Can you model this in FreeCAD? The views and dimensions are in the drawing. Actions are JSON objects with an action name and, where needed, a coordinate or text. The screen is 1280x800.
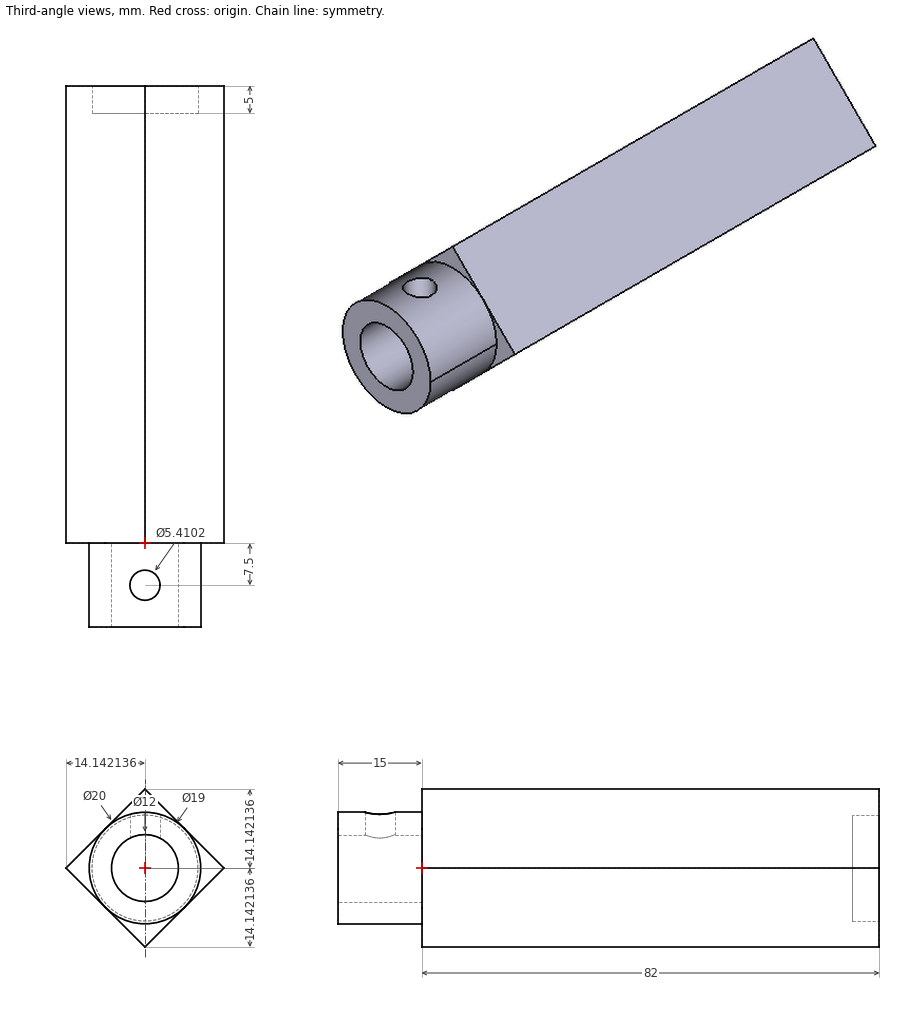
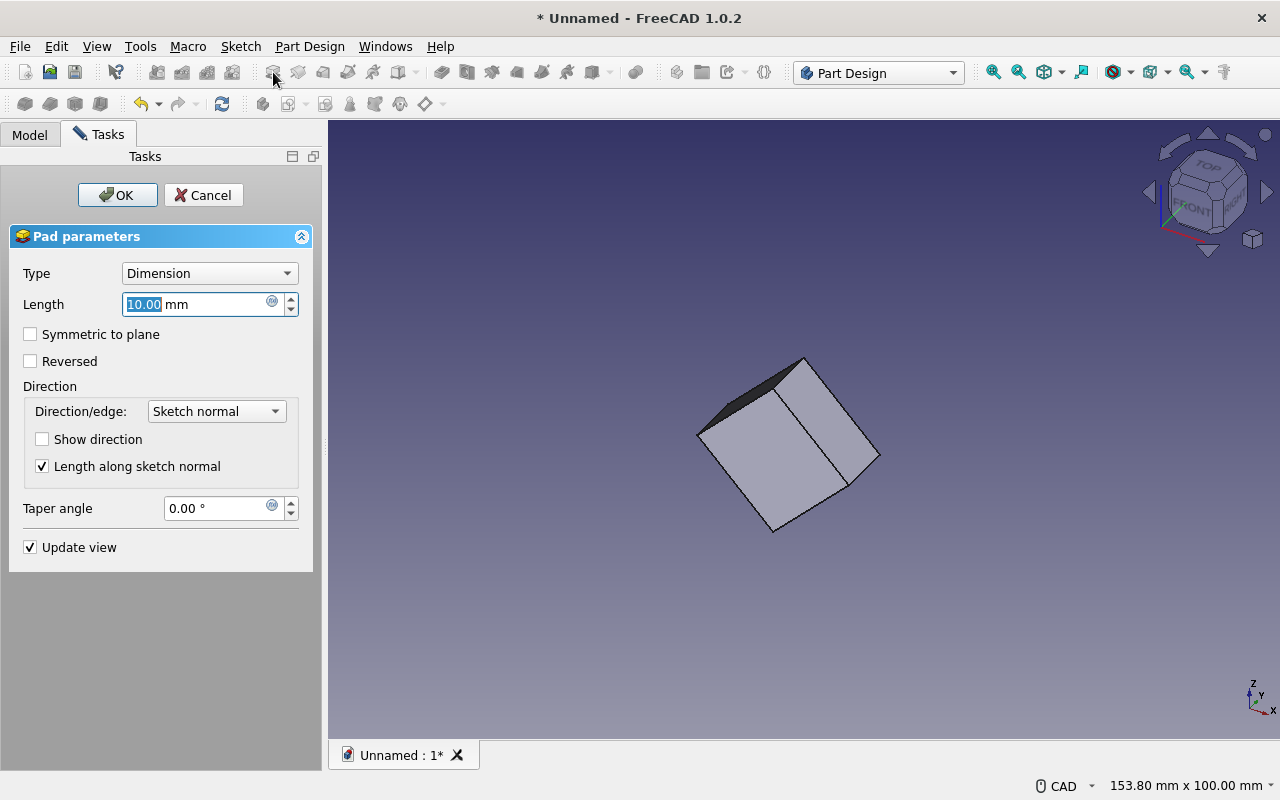
{"action": "type", "text": "82"}
{"action": "key", "text": "Tab"}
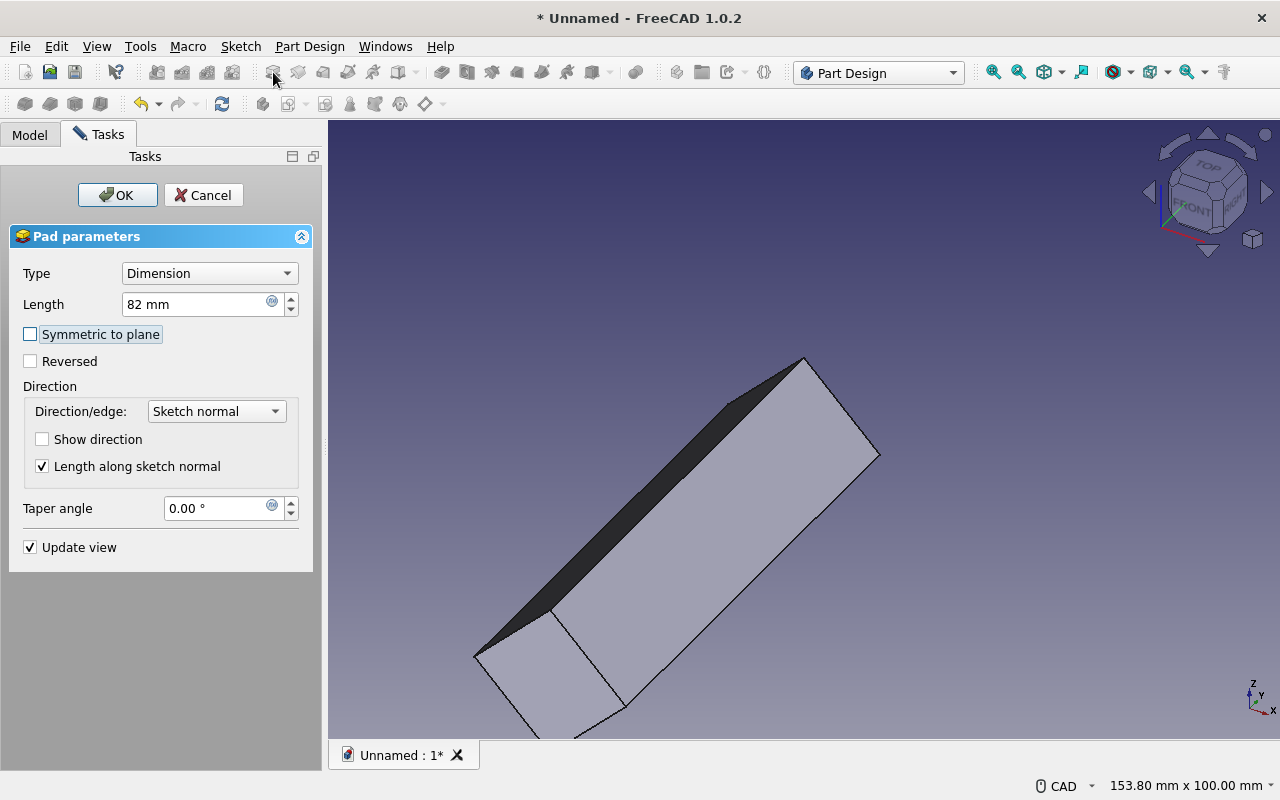
{"action": "left_click", "coordinate": [31, 361]}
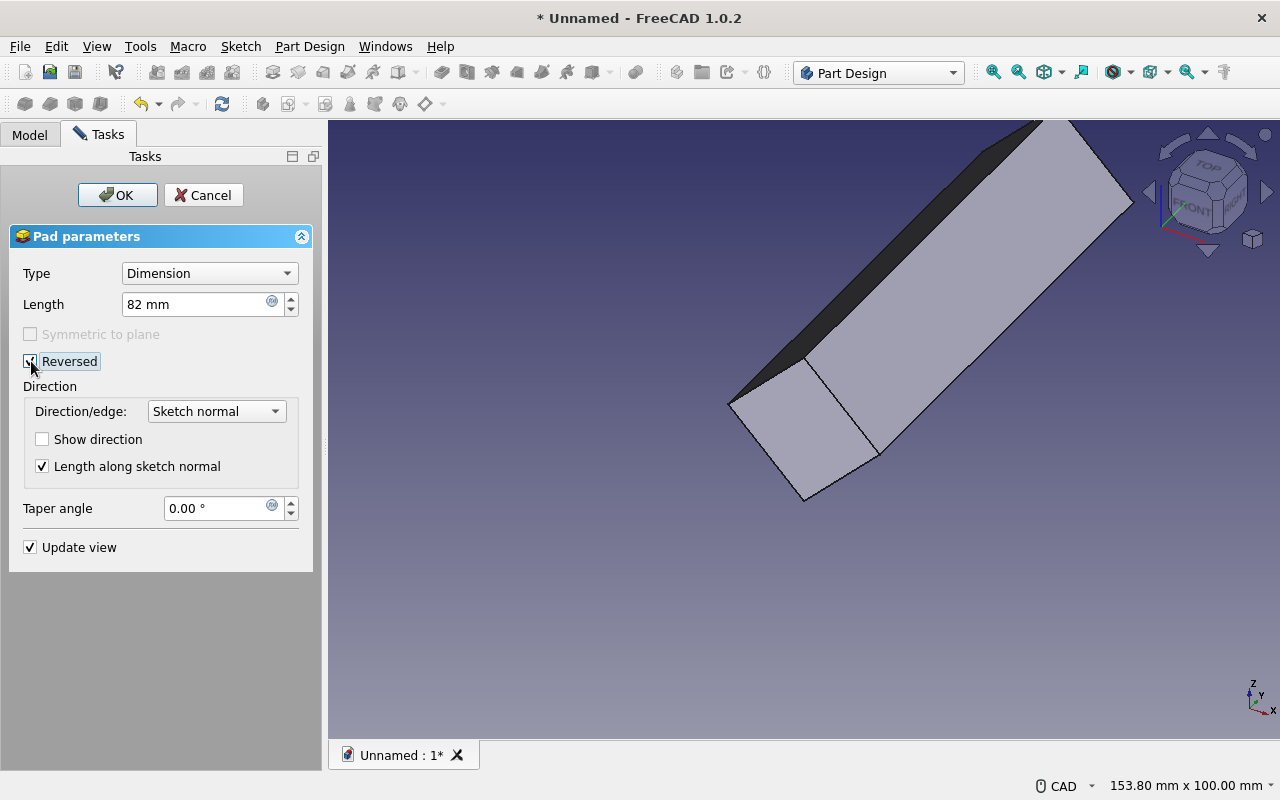
{"action": "left_click", "coordinate": [118, 195]}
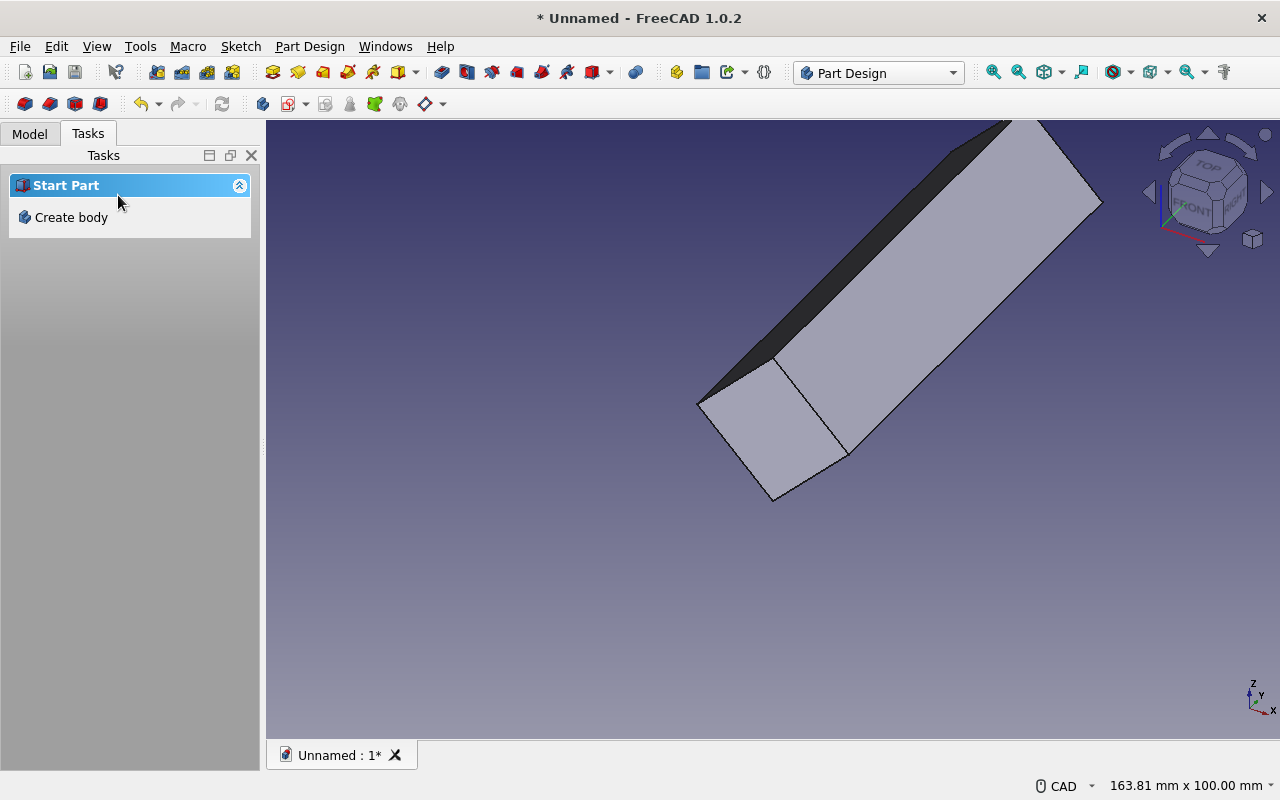
{"action": "key", "text": "v f"}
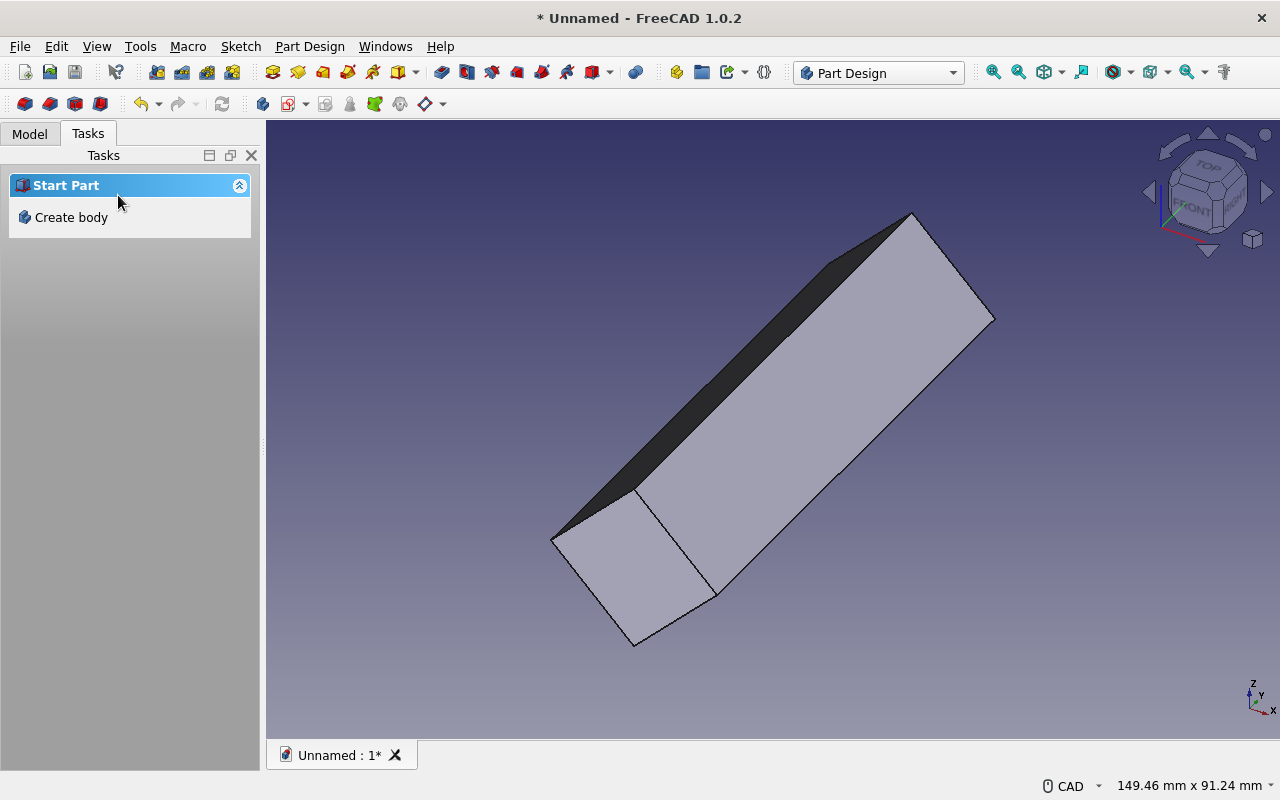
{"action": "key", "text": "4"}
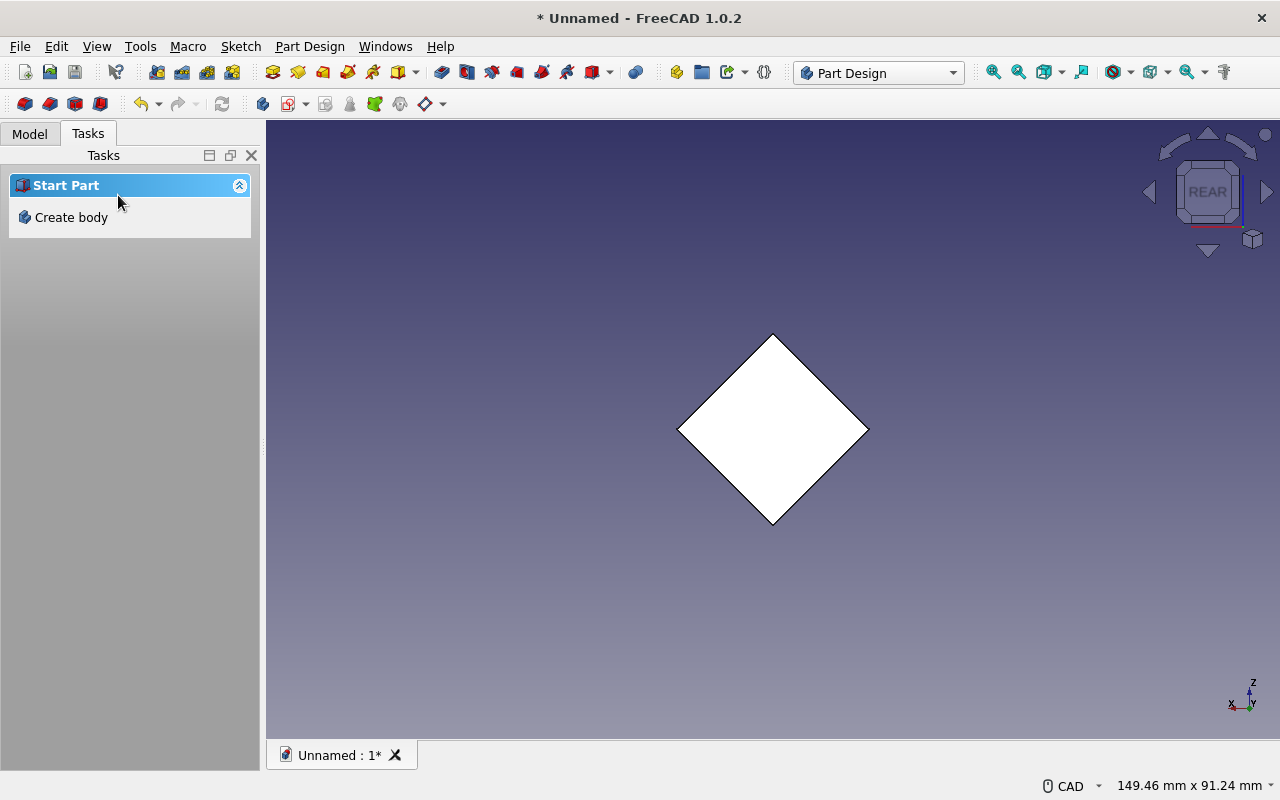
{"action": "key", "text": "v f"}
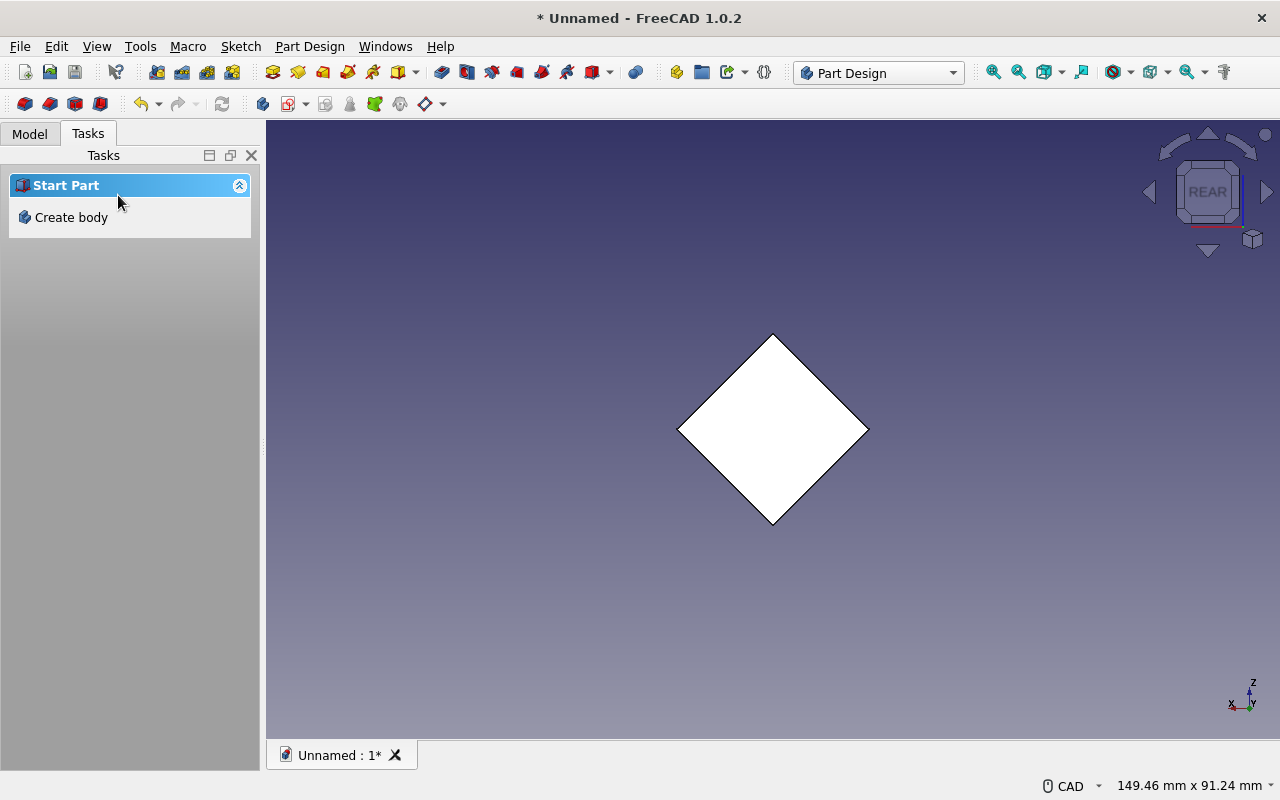
{"action": "left_click", "coordinate": [773, 429]}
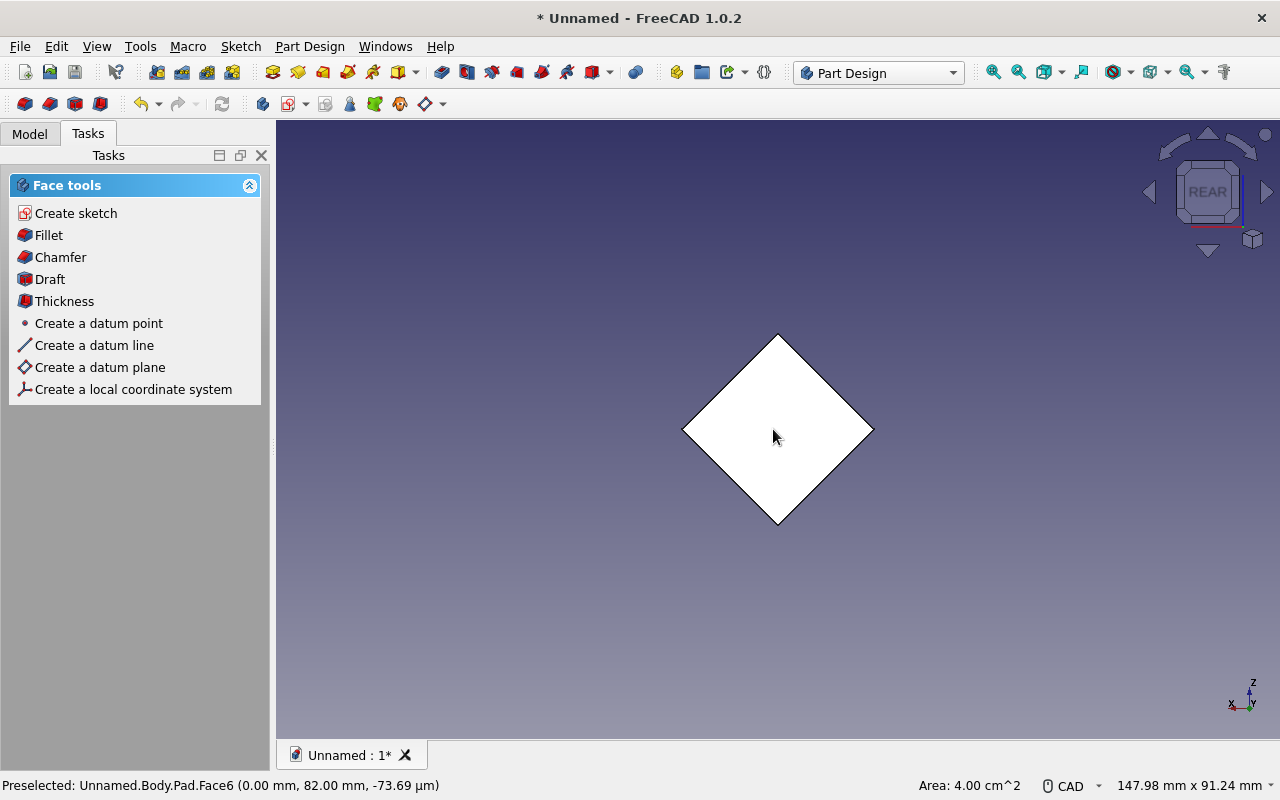
{"action": "left_click", "coordinate": [288, 104]}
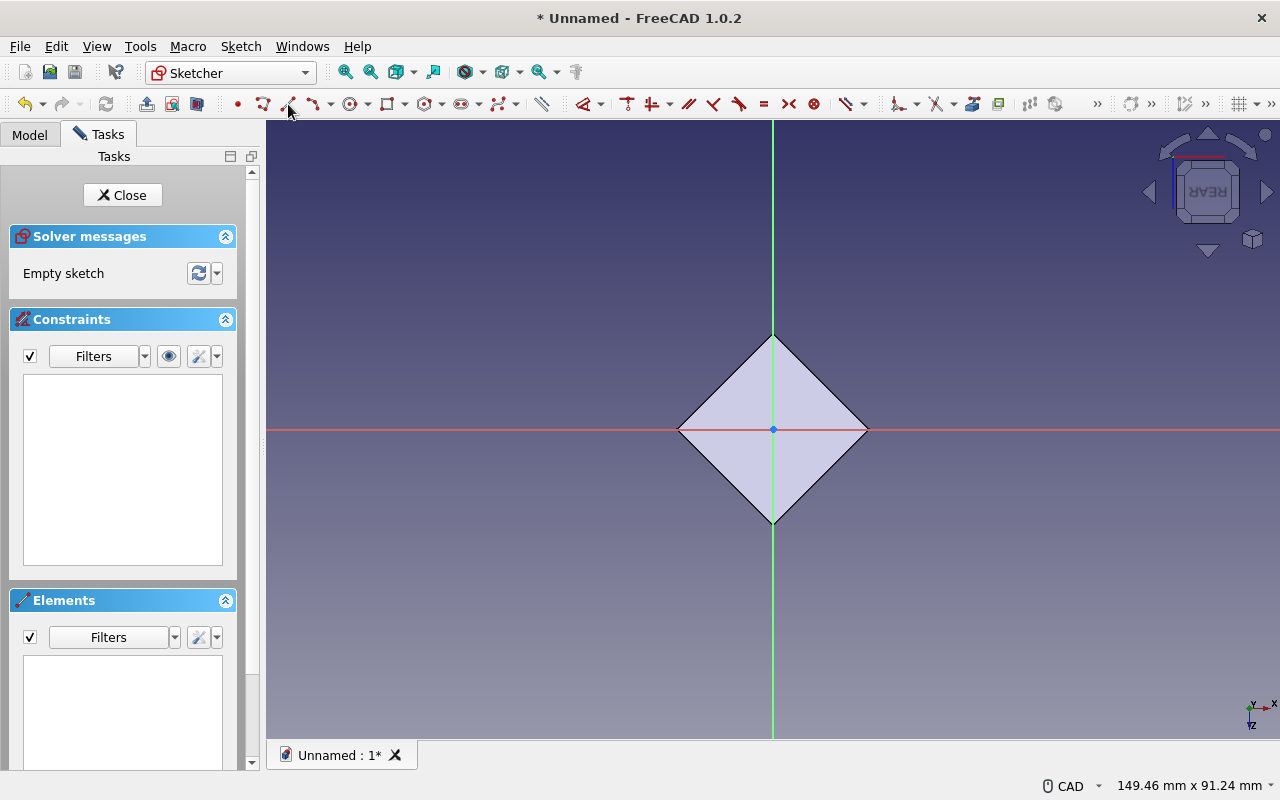
{"action": "scroll", "coordinate": [803, 429], "scroll_direction": "up", "scroll_amount": 6}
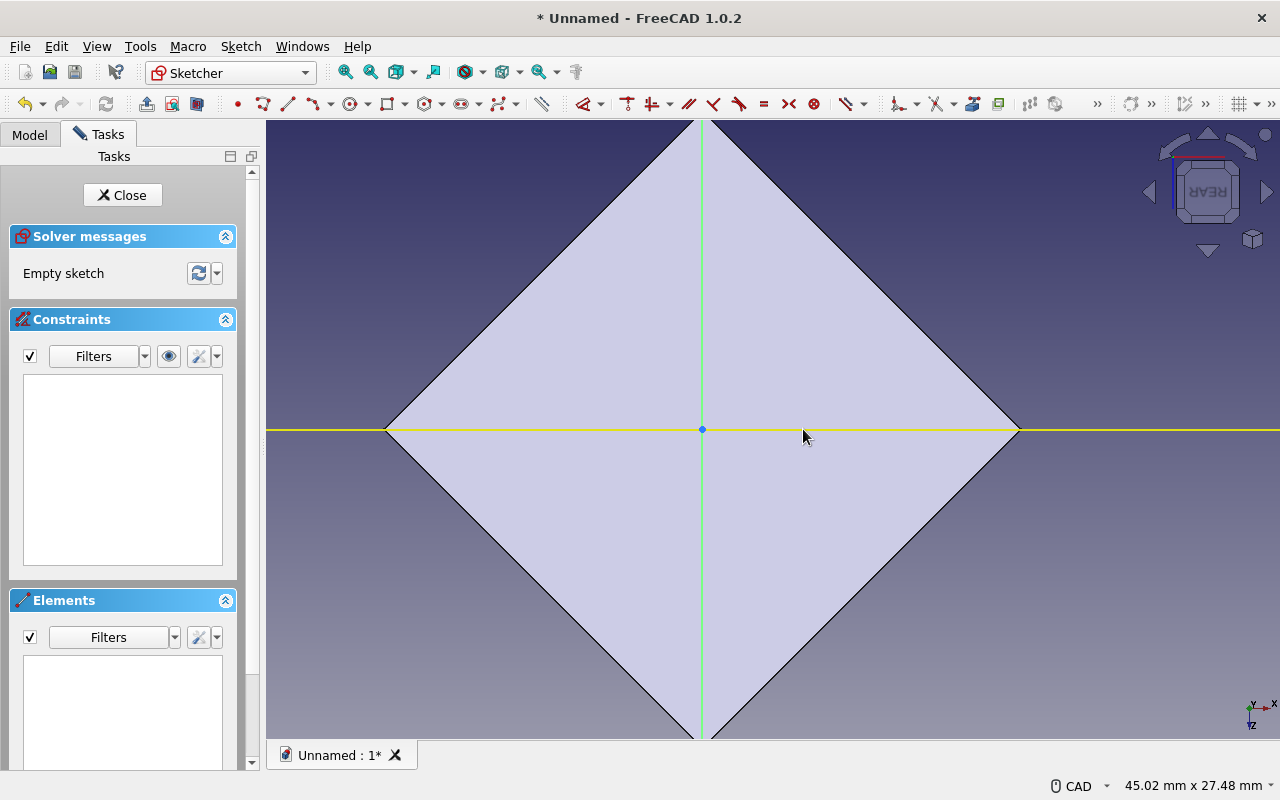
{"action": "left_click", "coordinate": [350, 104]}